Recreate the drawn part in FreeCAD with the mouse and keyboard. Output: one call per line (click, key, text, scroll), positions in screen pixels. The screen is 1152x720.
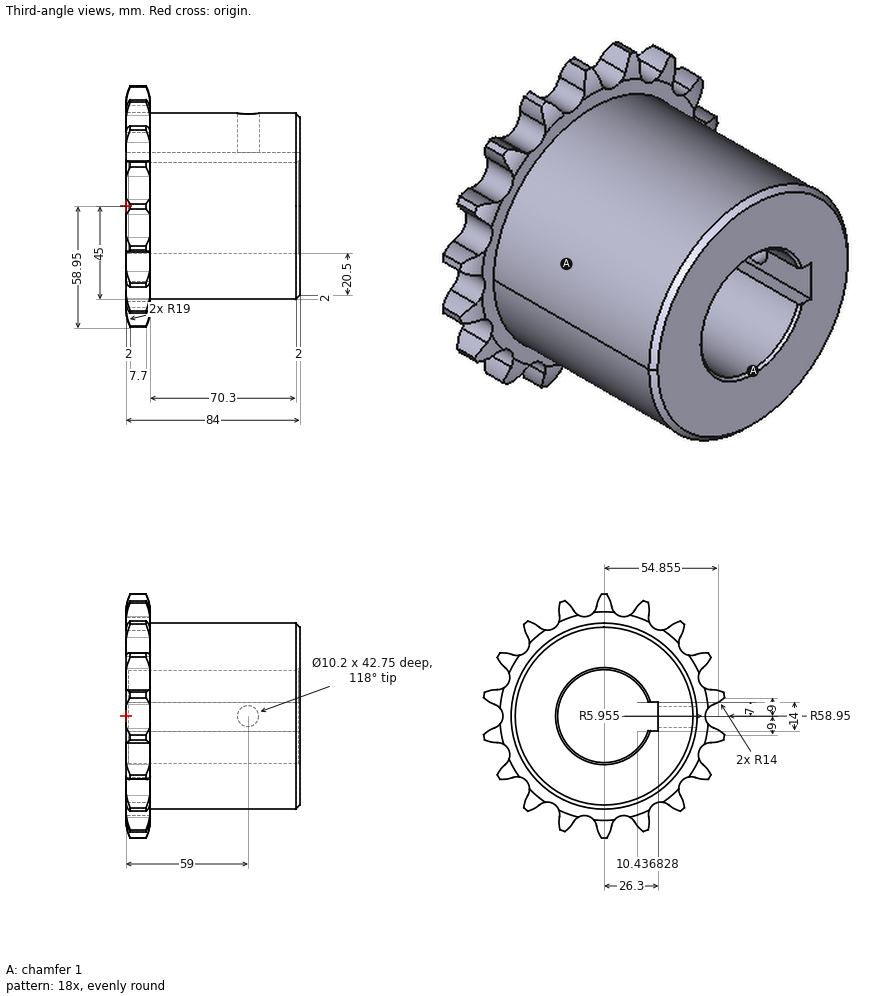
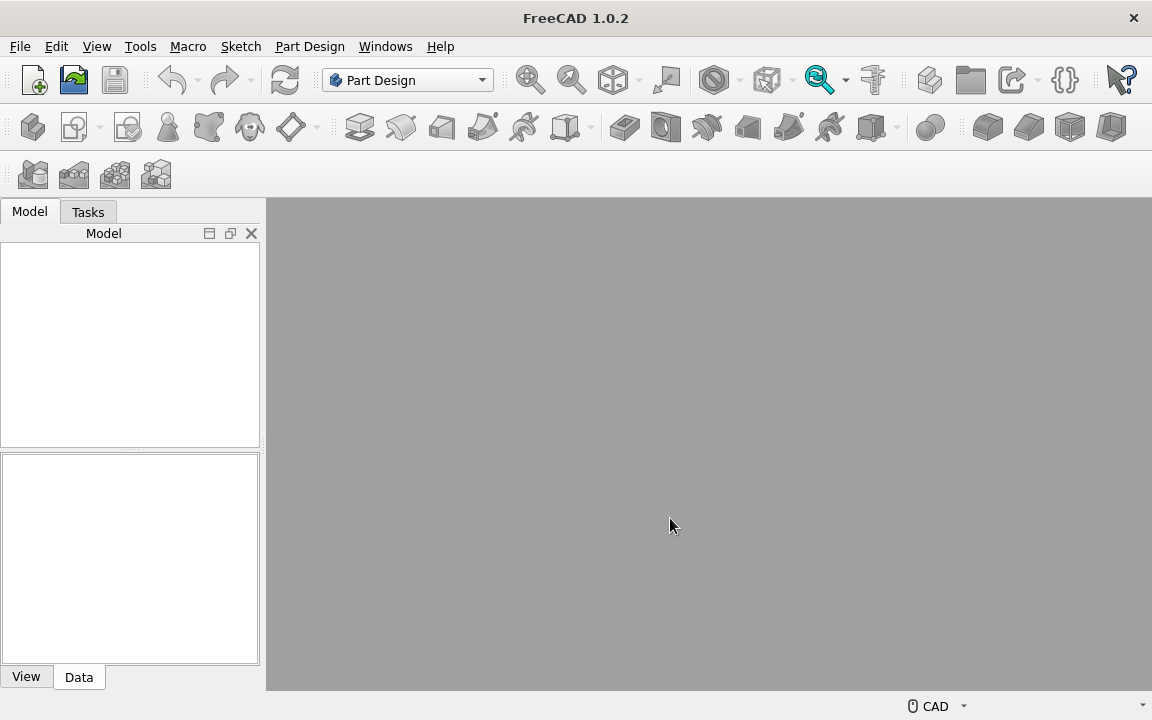
click(33, 80)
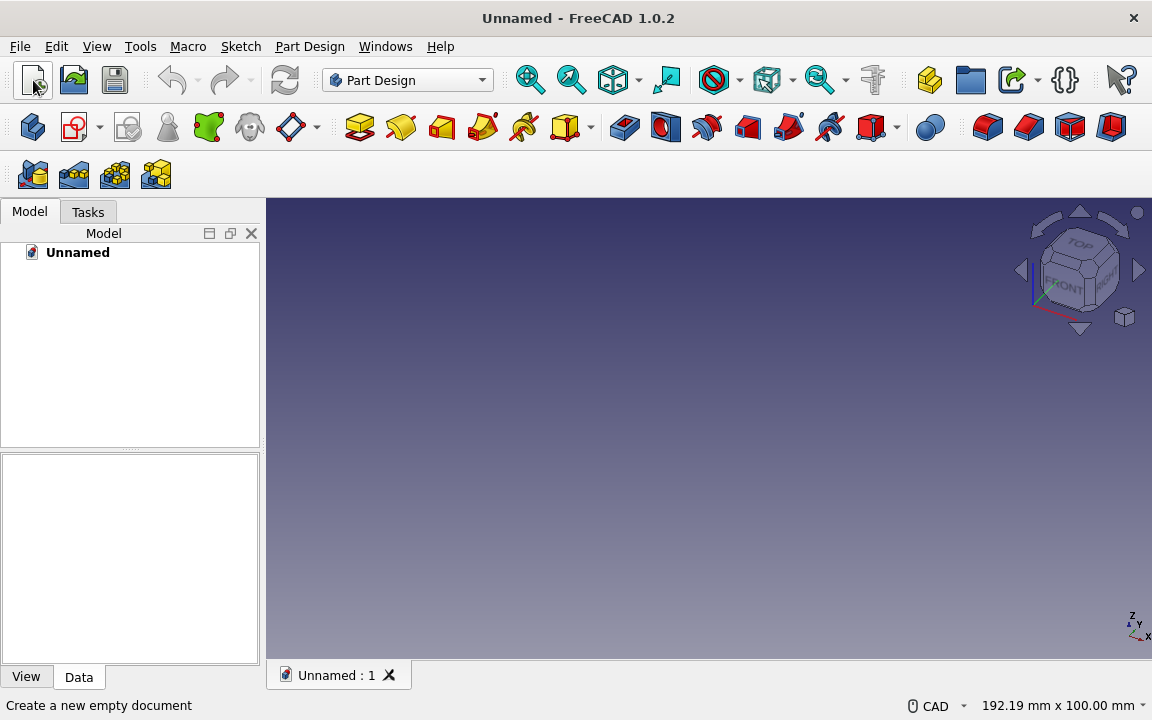
click(74, 128)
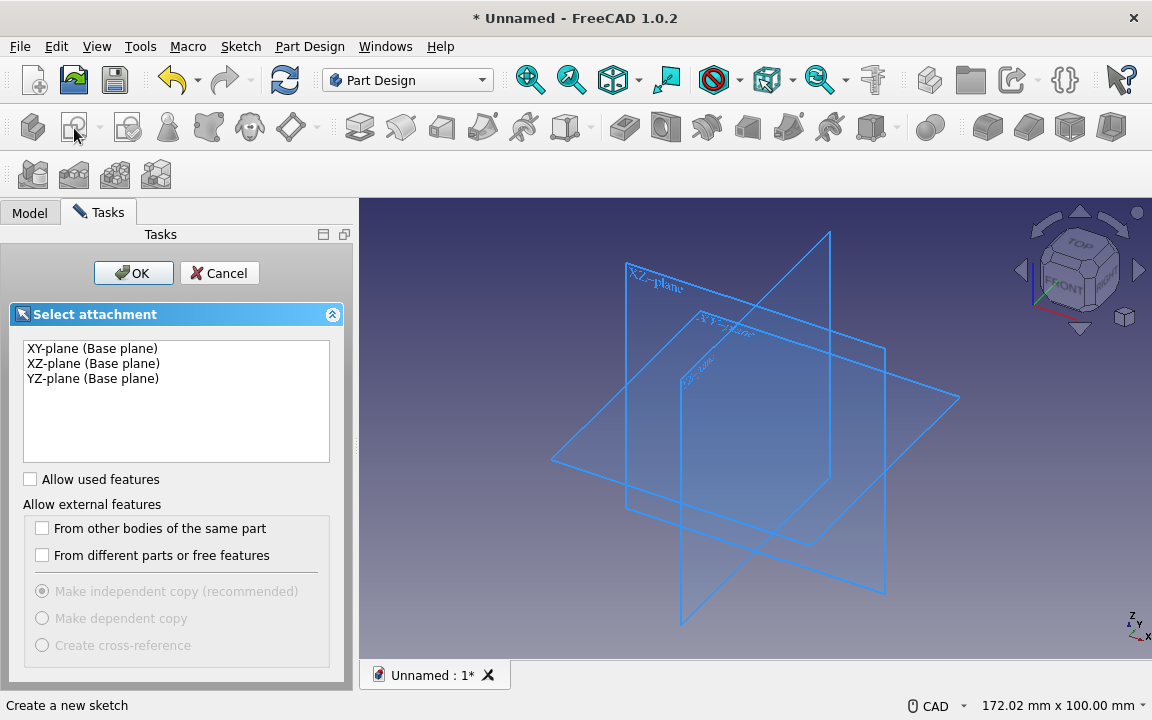
click(84, 348)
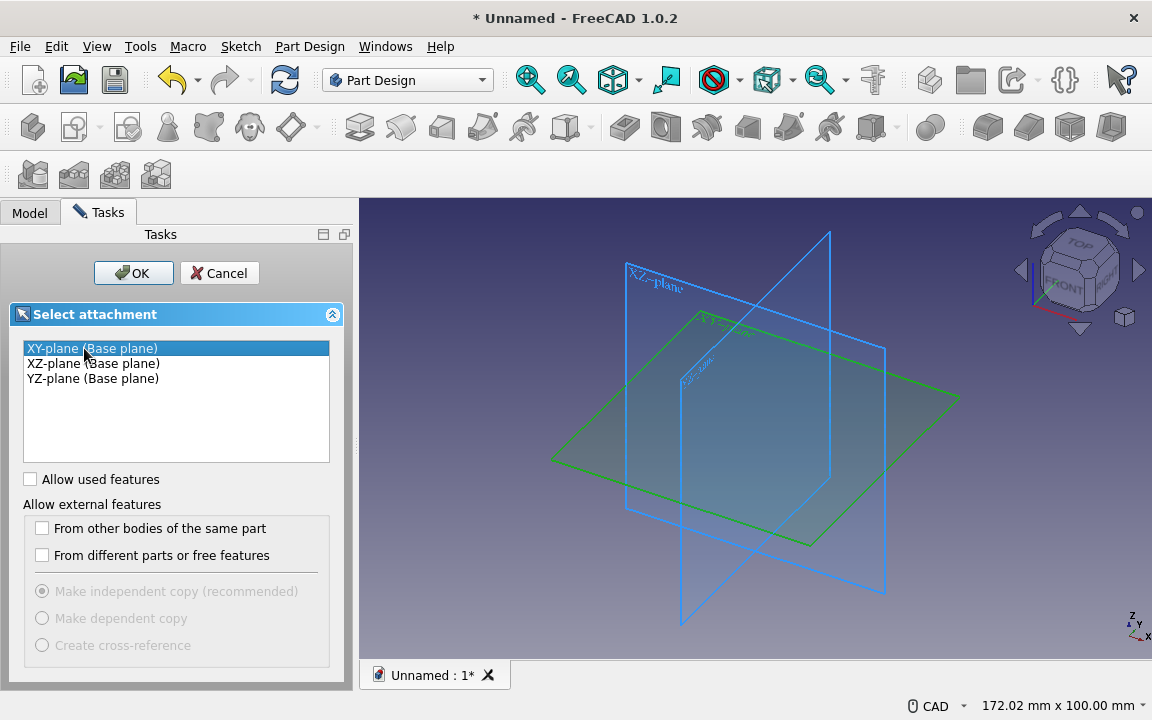
click(134, 273)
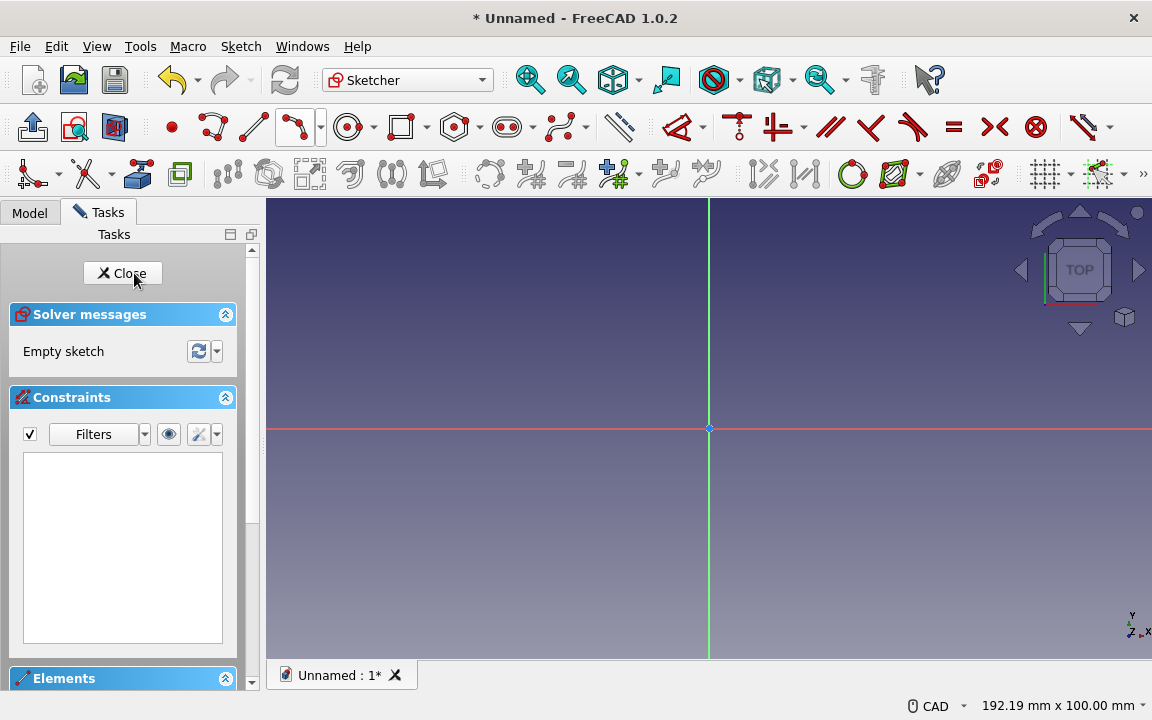
scroll(294, 226, down, 2)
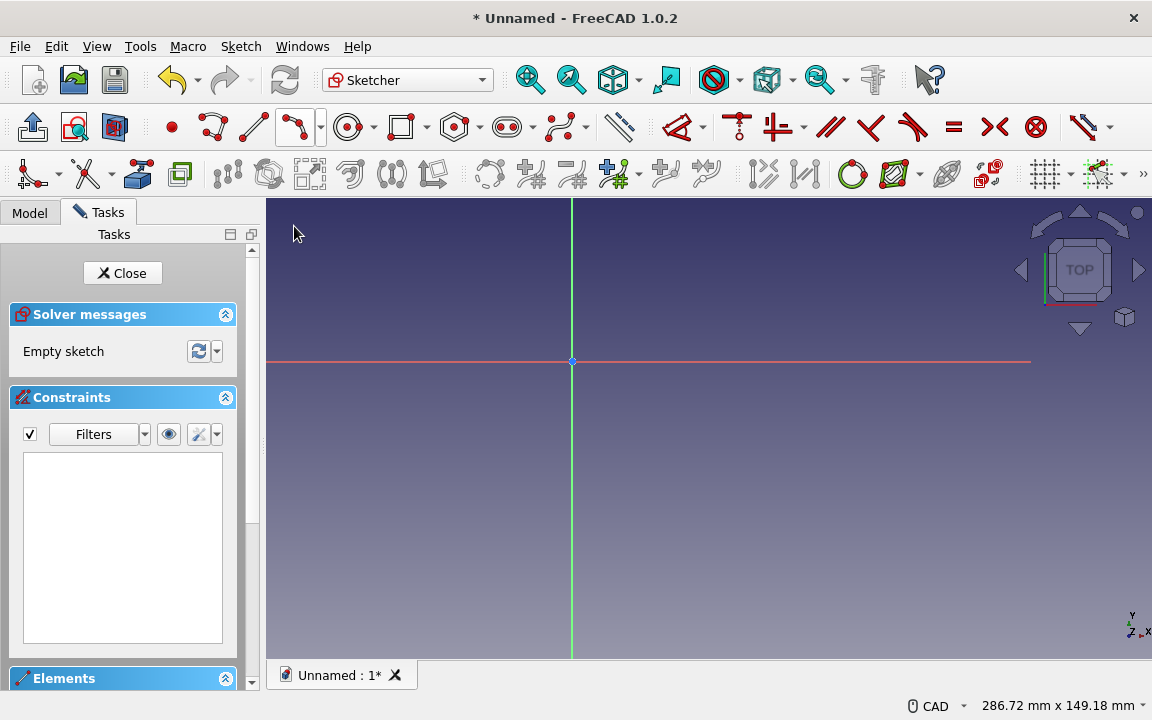
scroll(827, 502, up, 2)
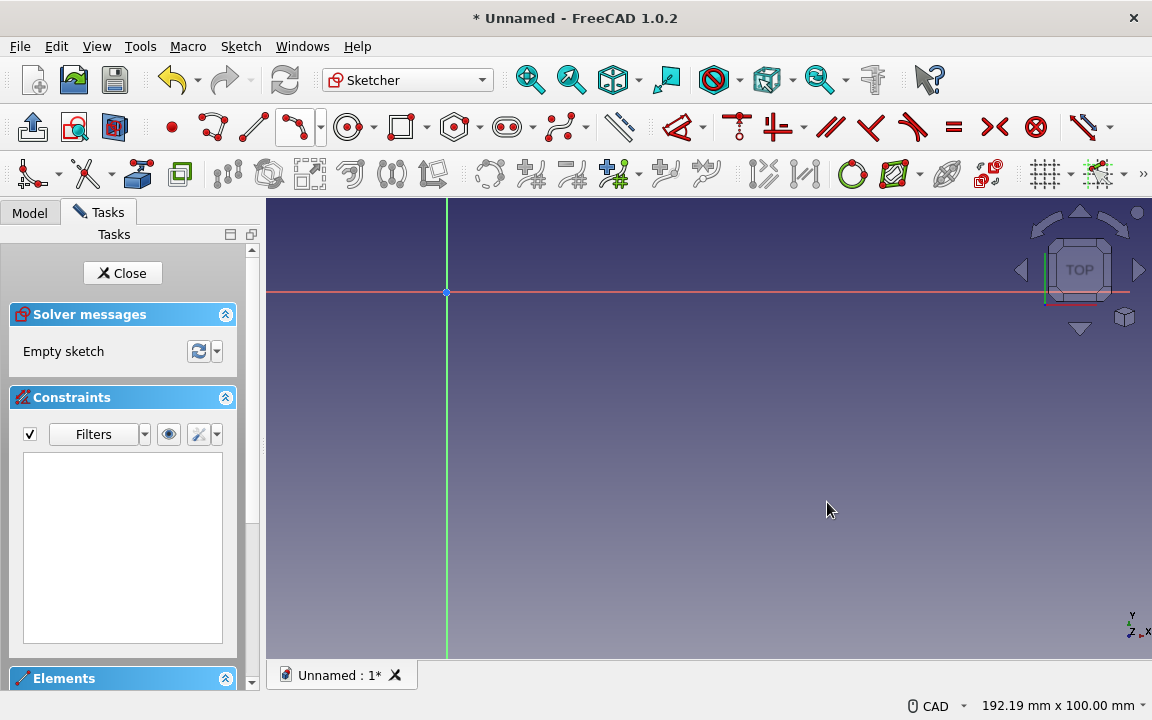
click(254, 128)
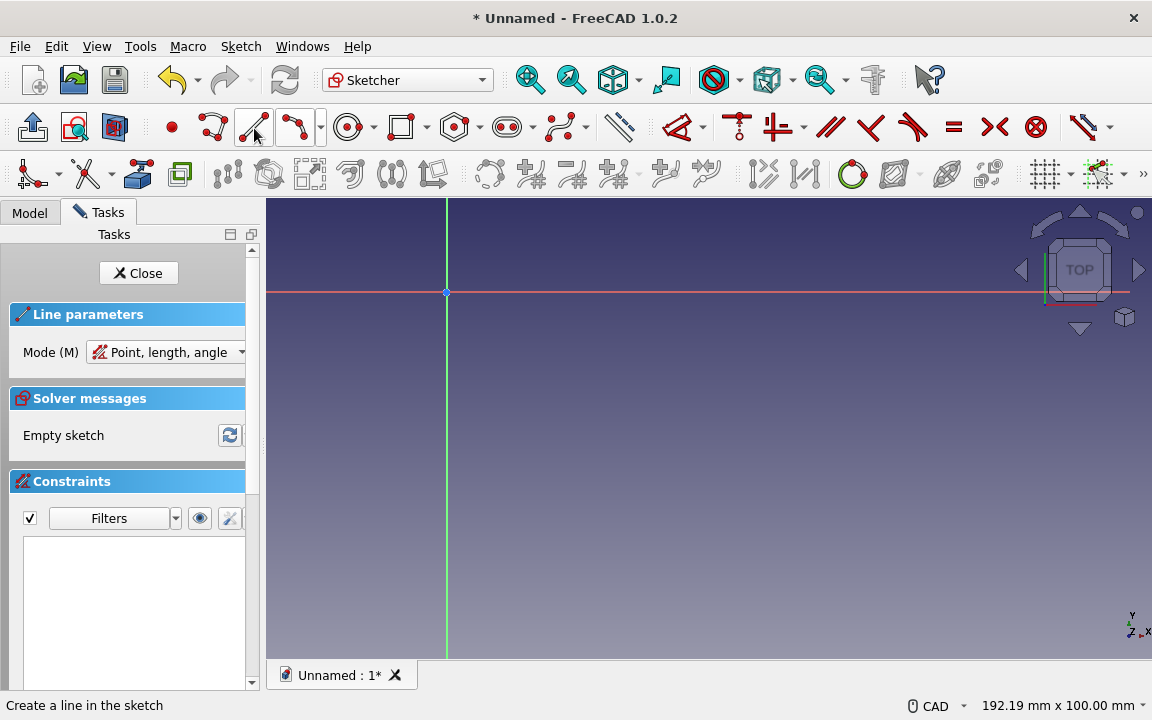
scroll(456, 564, up, 3)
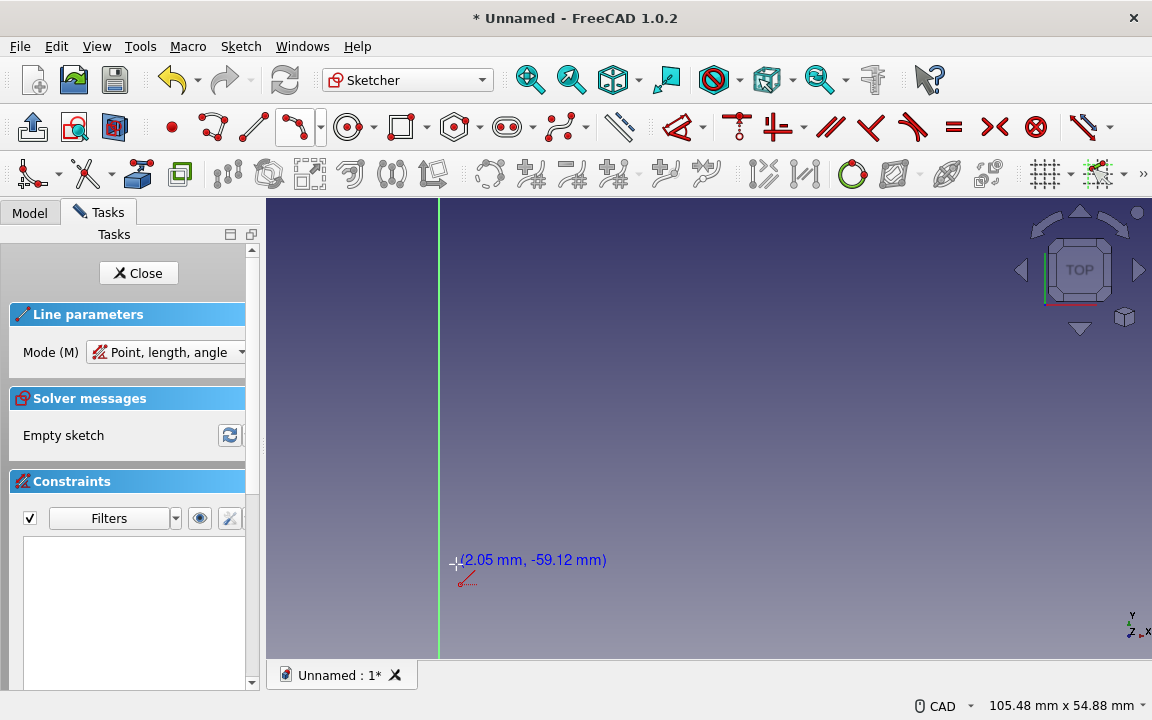
click(455, 564)
click(520, 564)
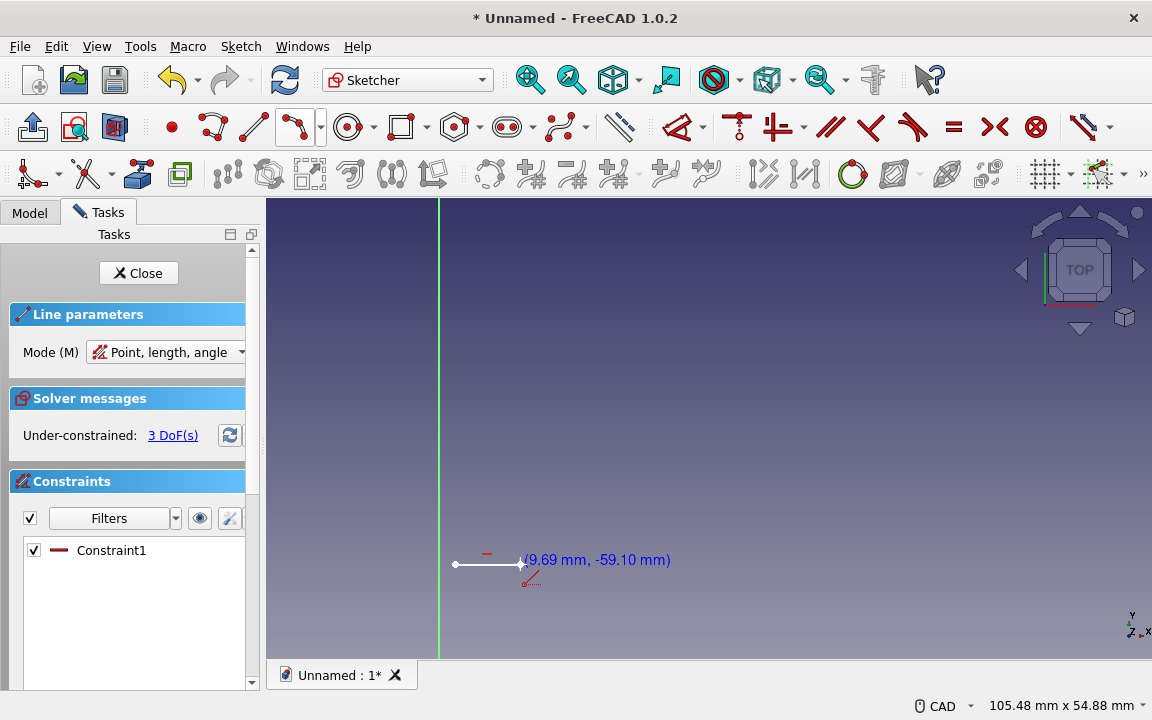
click(213, 128)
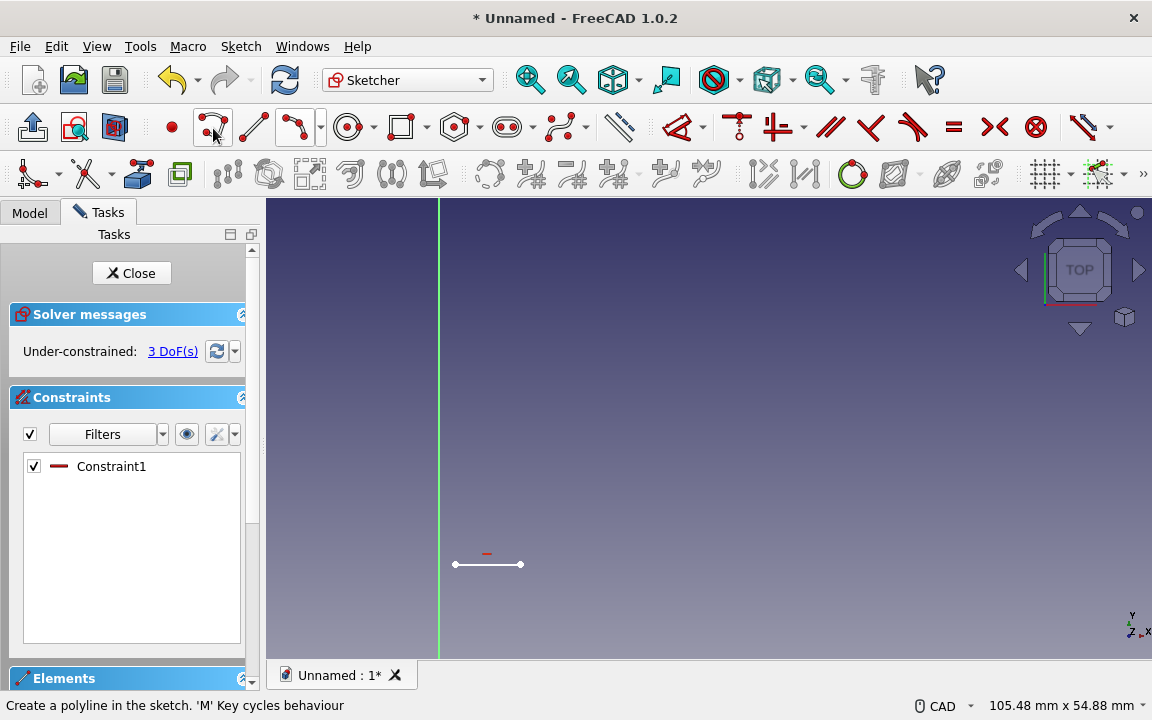
click(537, 492)
click(537, 447)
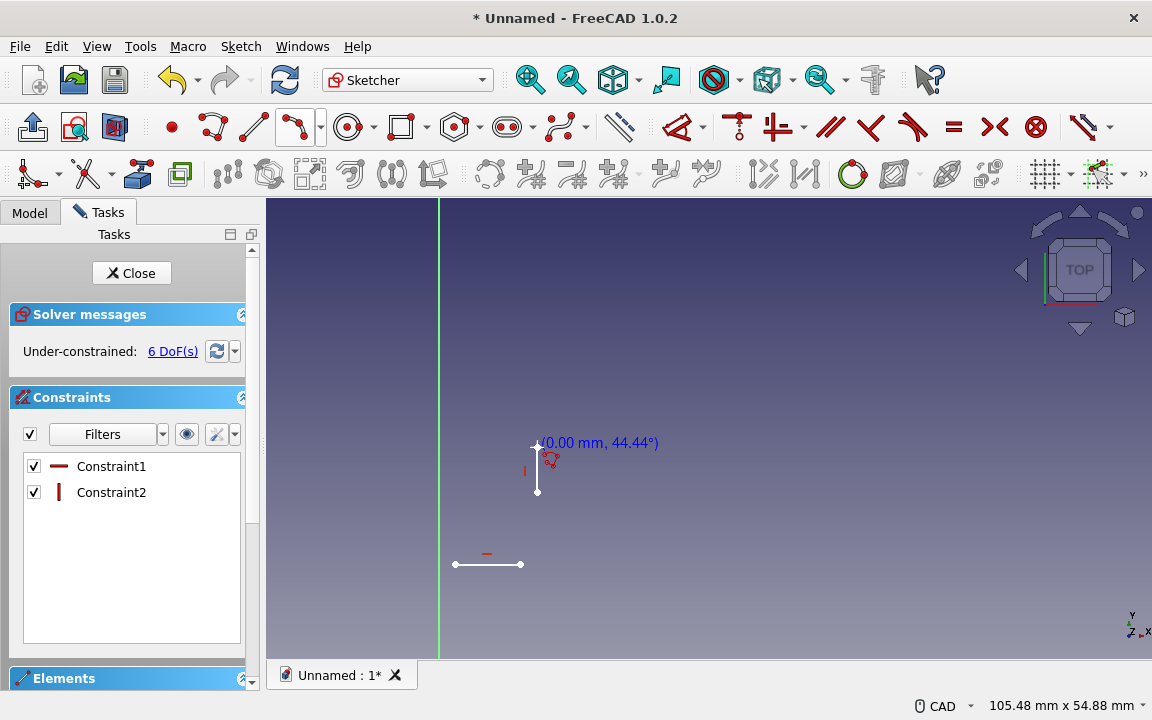
scroll(457, 565, down, 3)